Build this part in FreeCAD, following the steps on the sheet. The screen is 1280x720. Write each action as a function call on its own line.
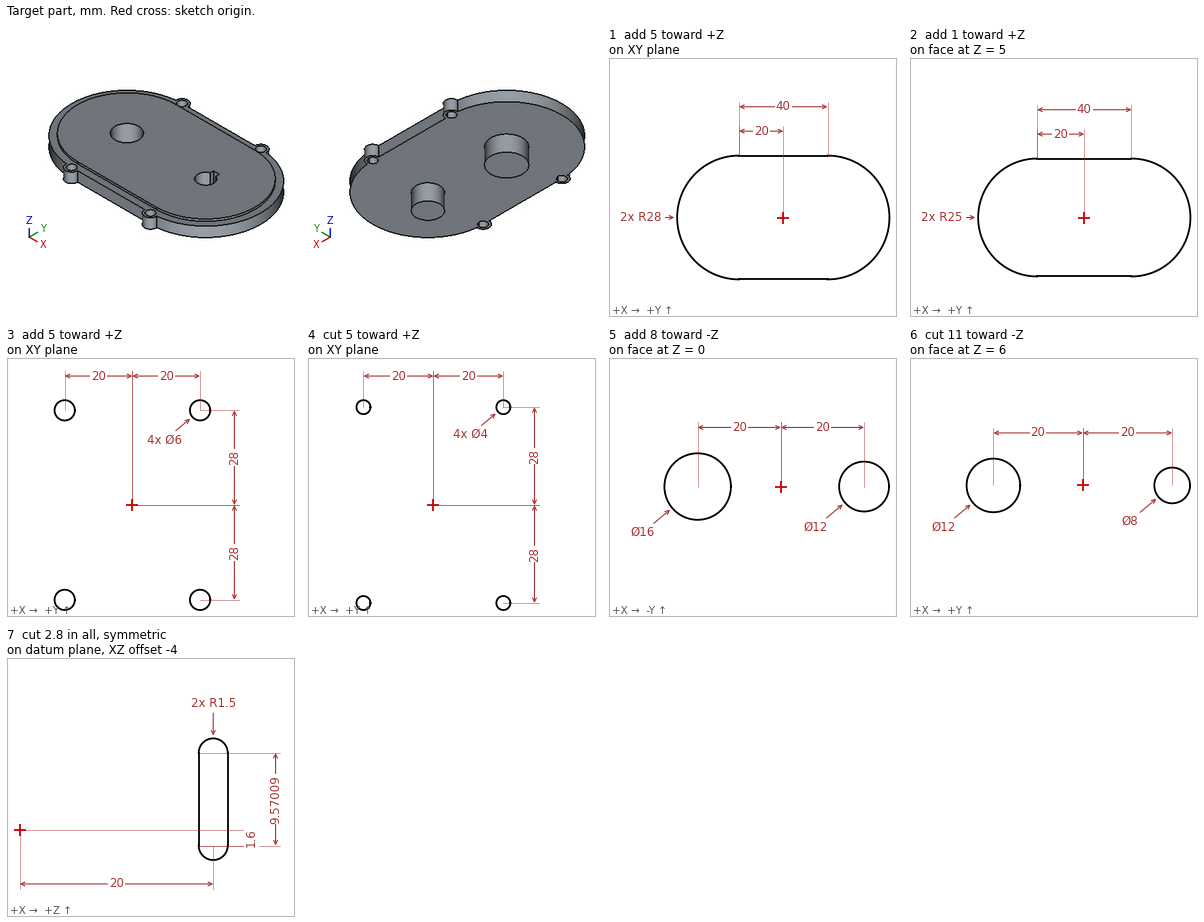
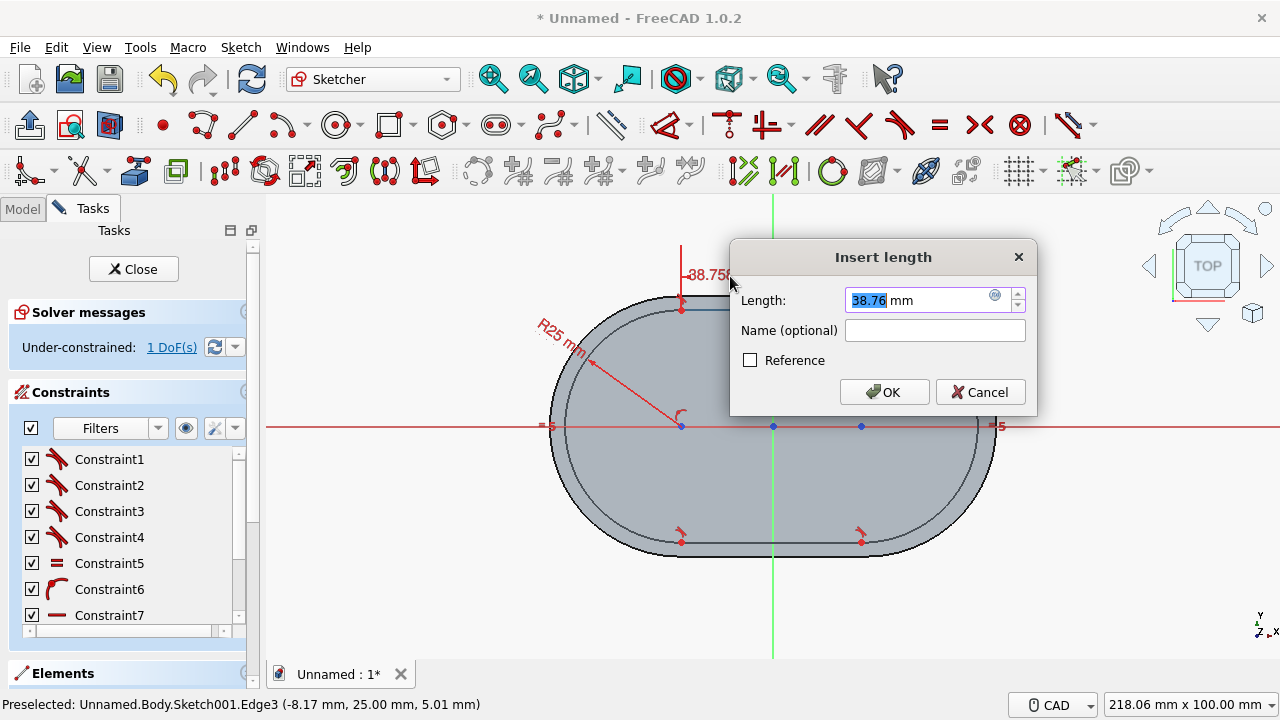
text(40)
key(Return)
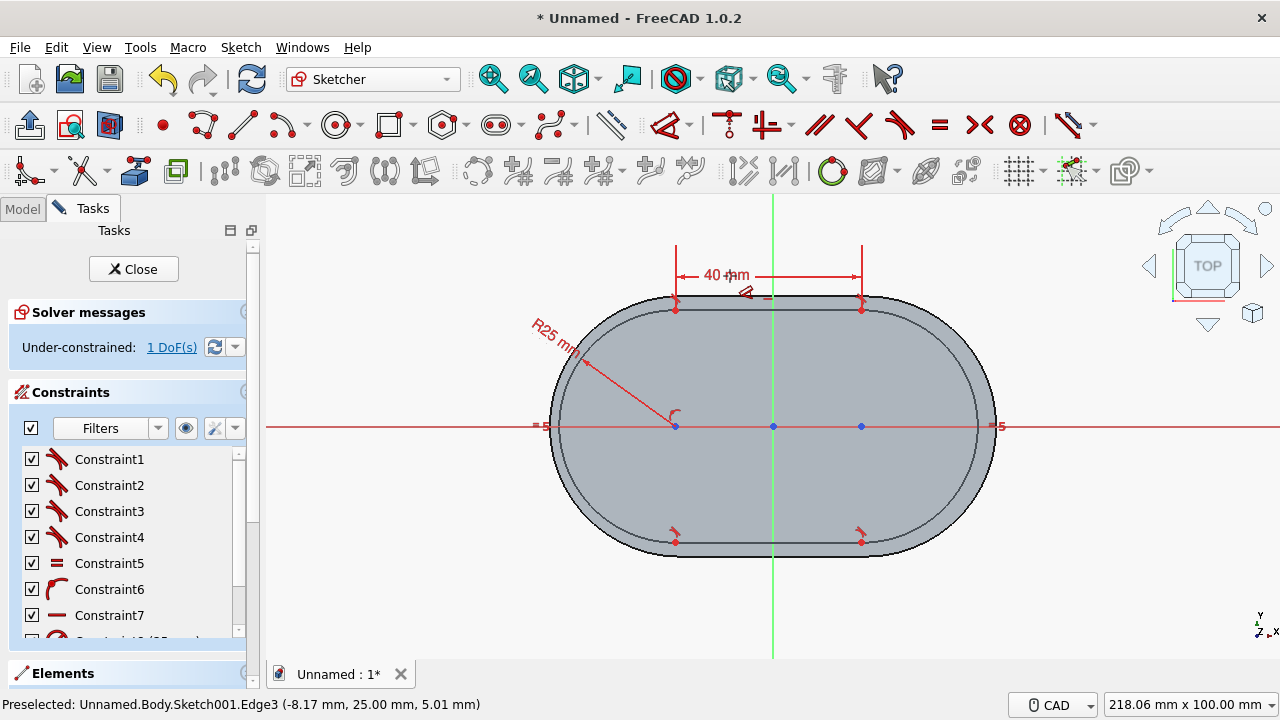
click(676, 310)
click(724, 460)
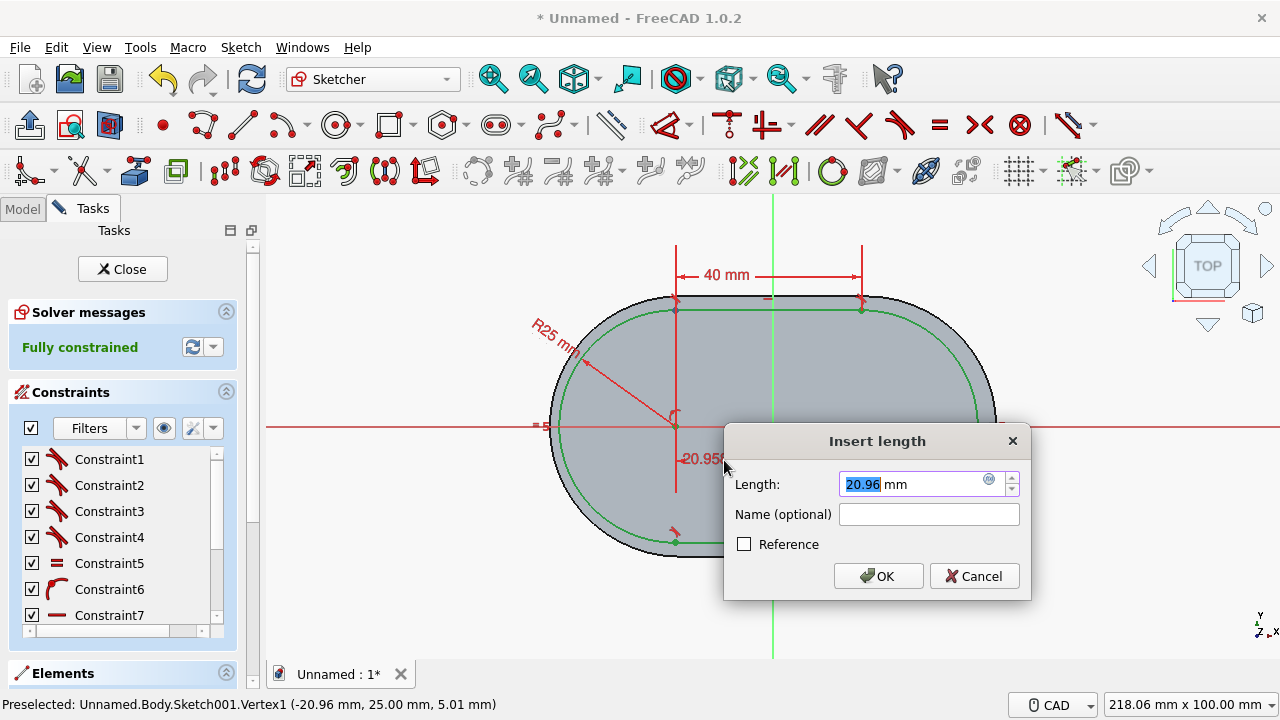
text(20)
key(Return)
key(Escape)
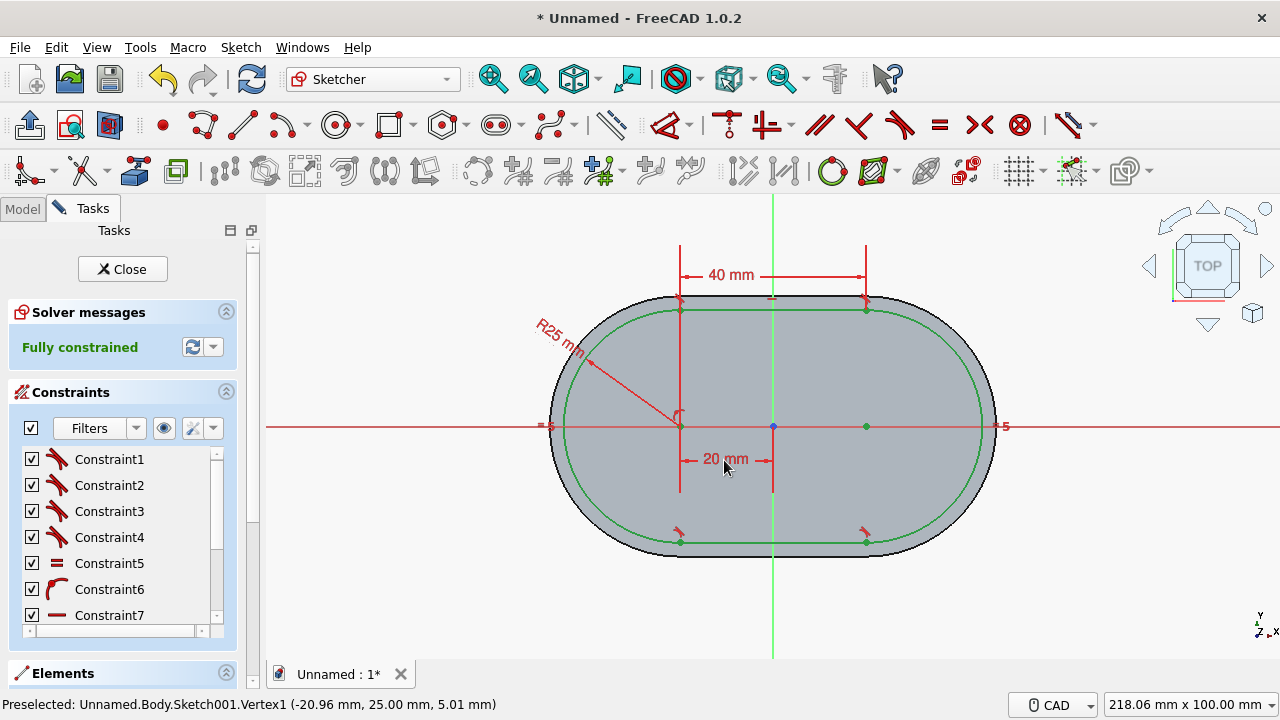
click(123, 269)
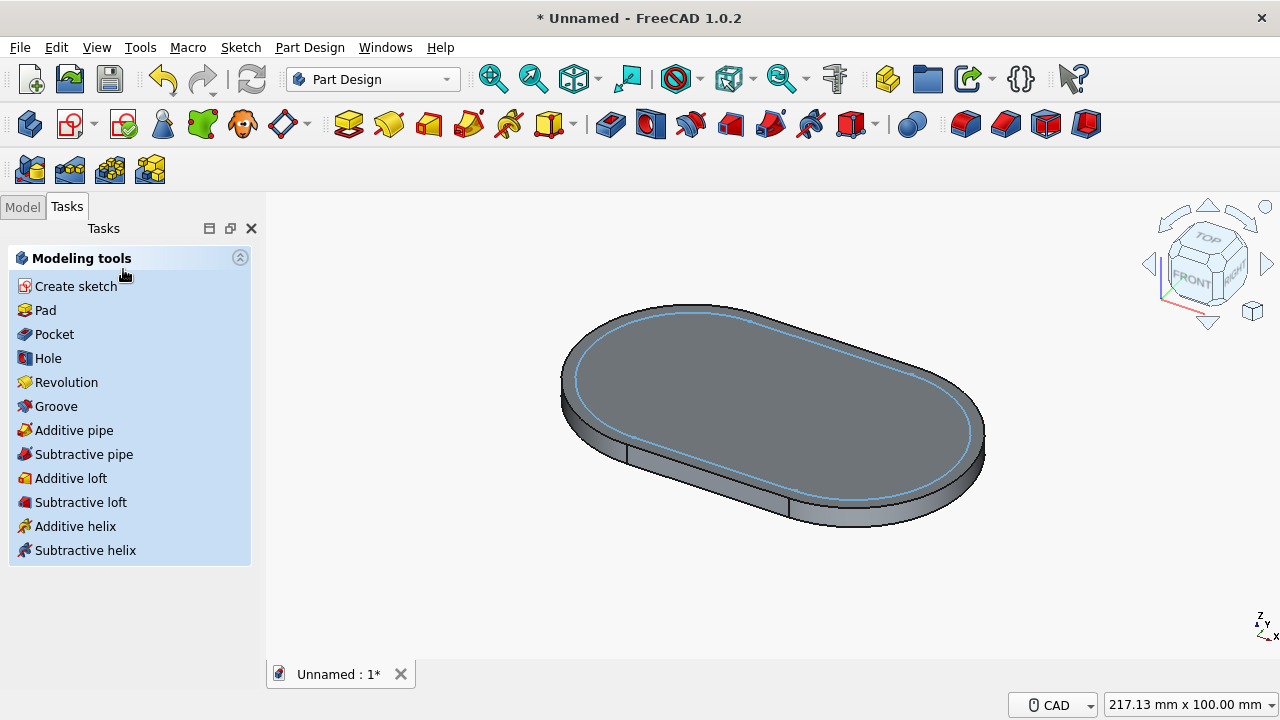
click(350, 124)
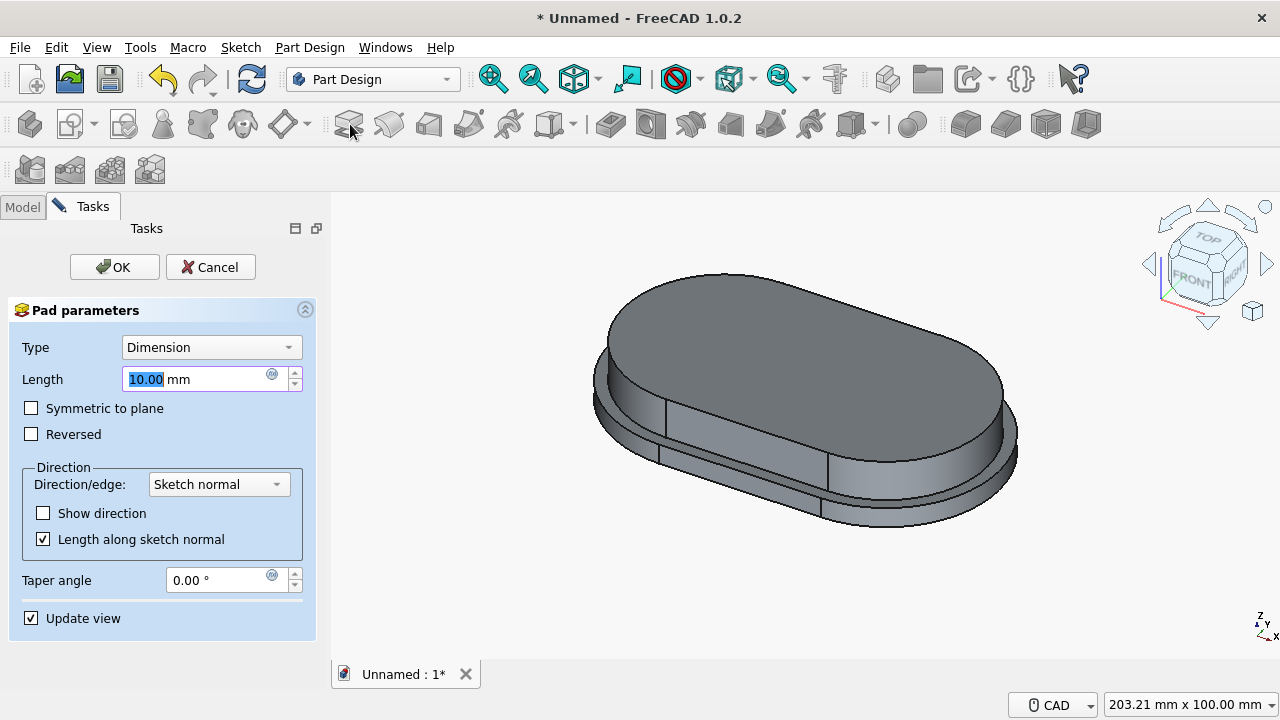
text(1)
key(Tab)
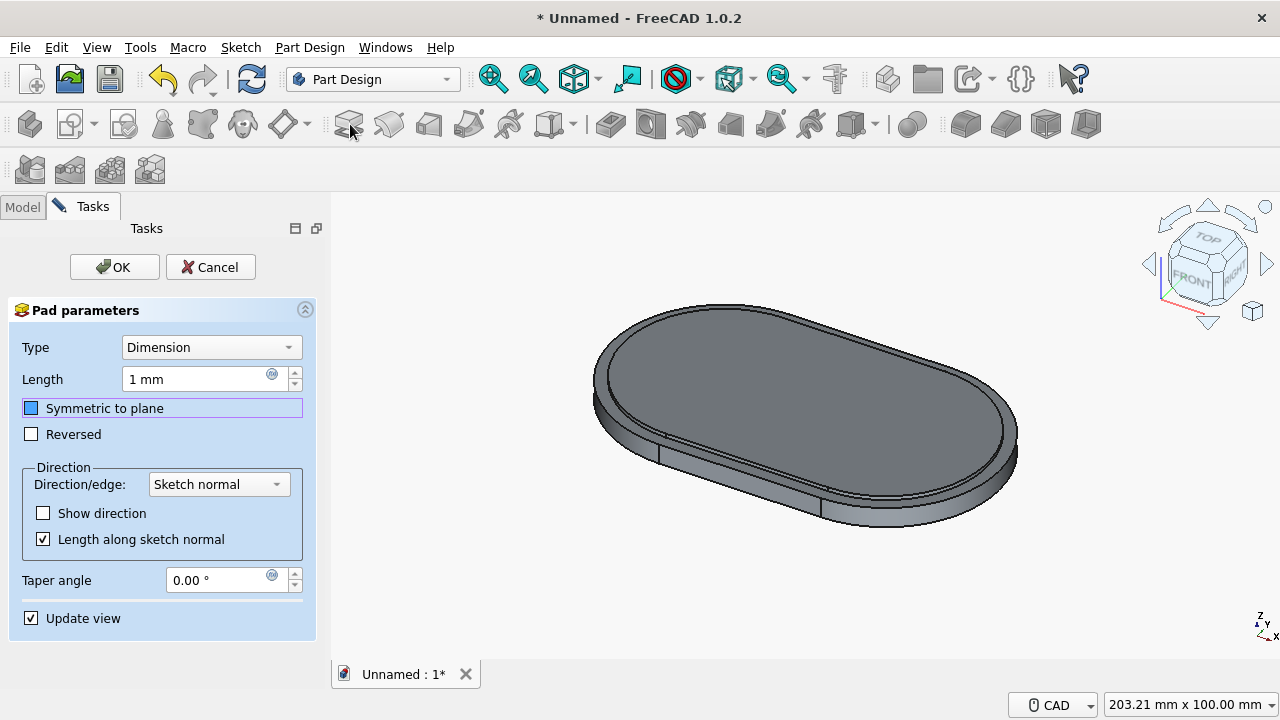
click(115, 267)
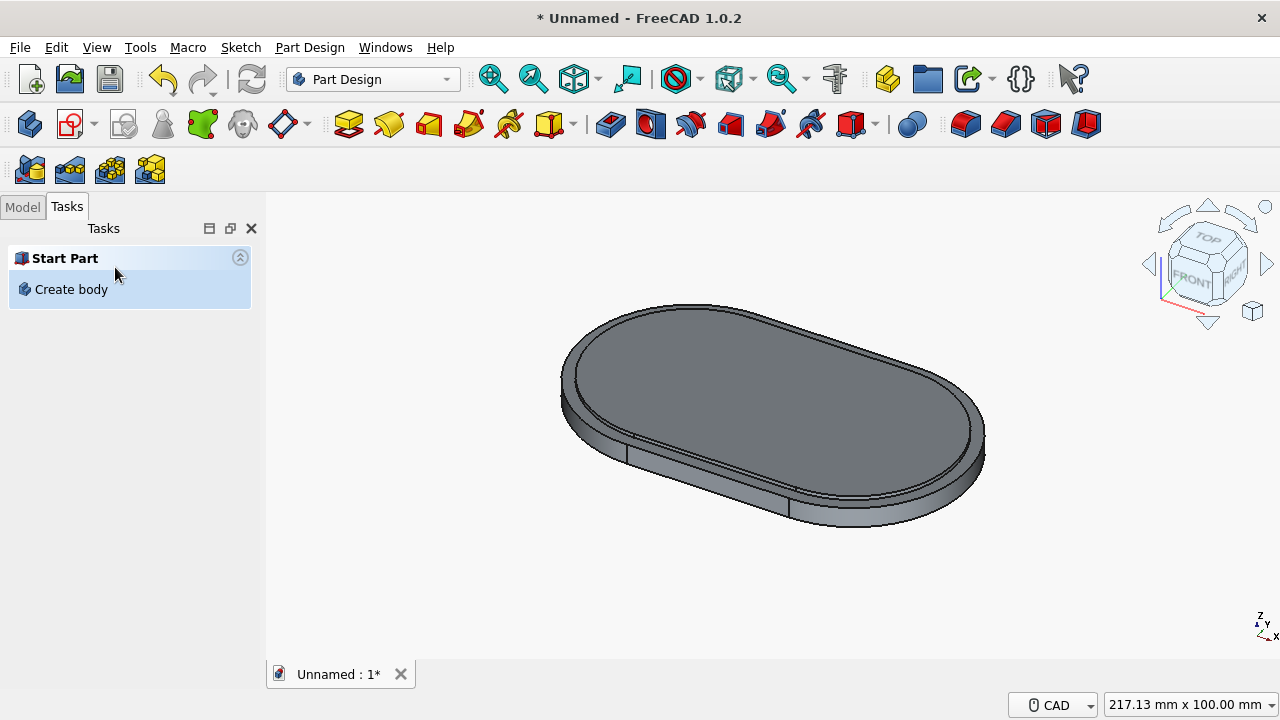
click(70, 124)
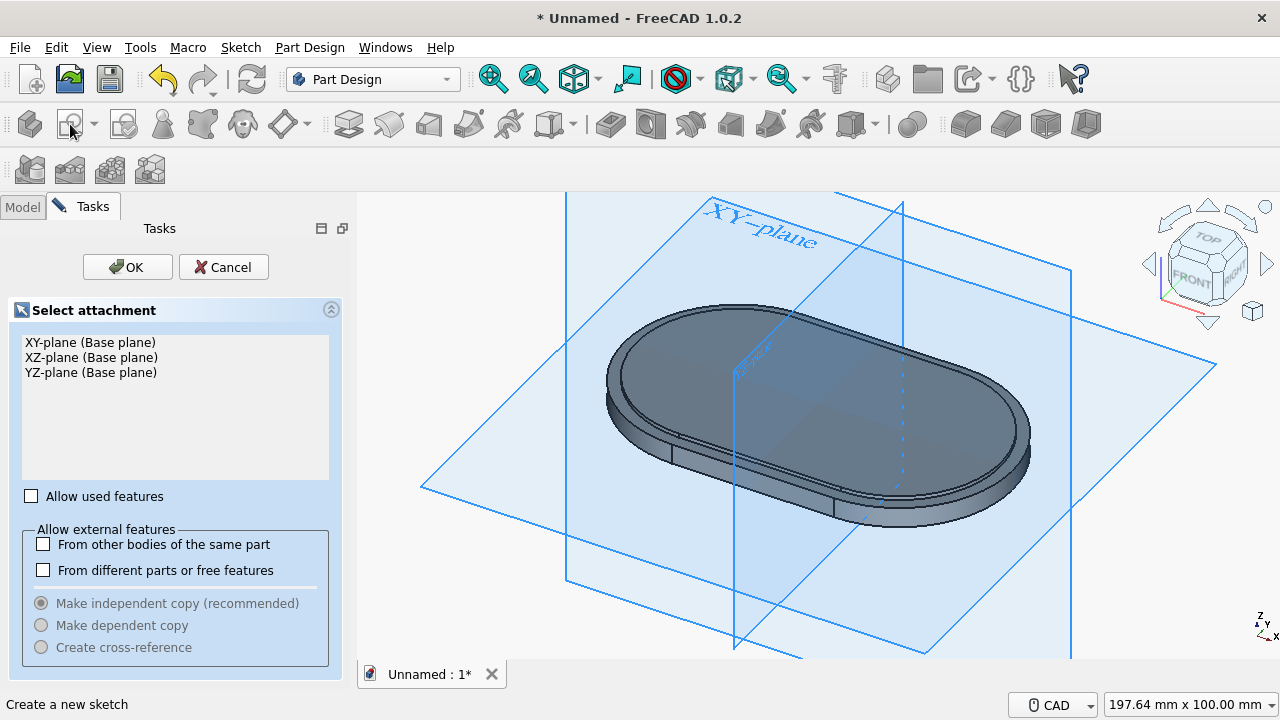
click(82, 342)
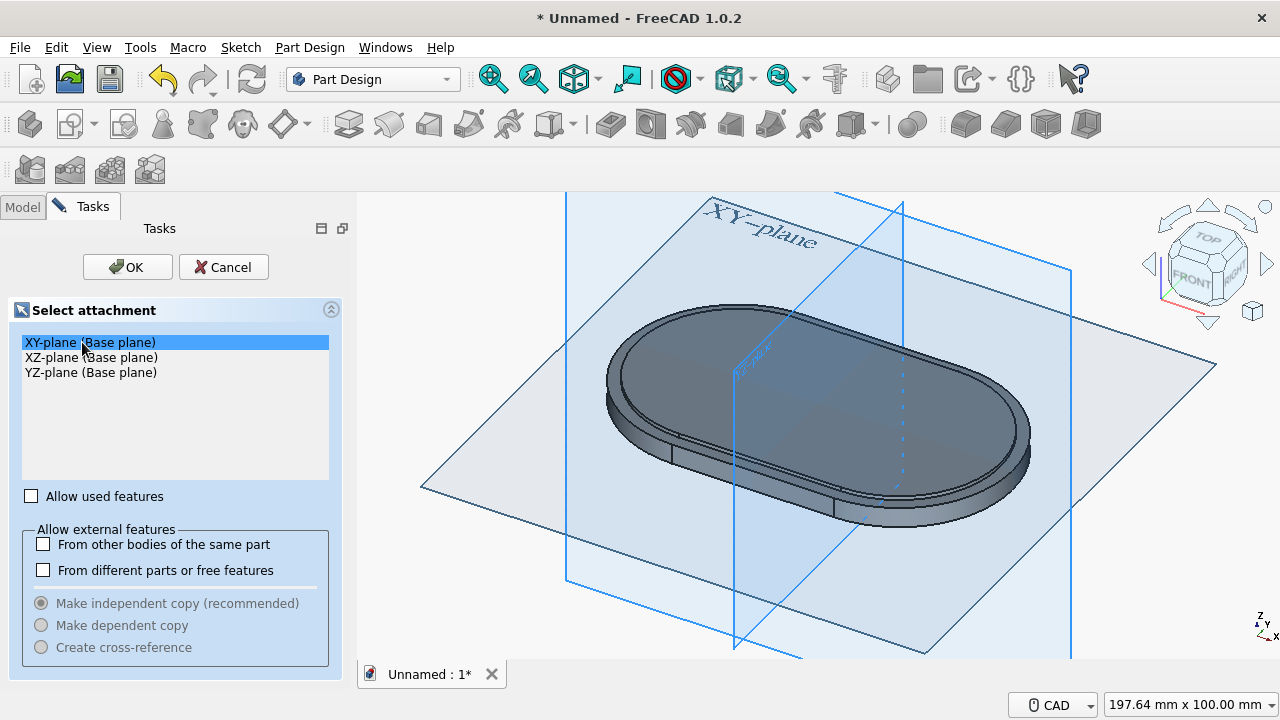
click(128, 267)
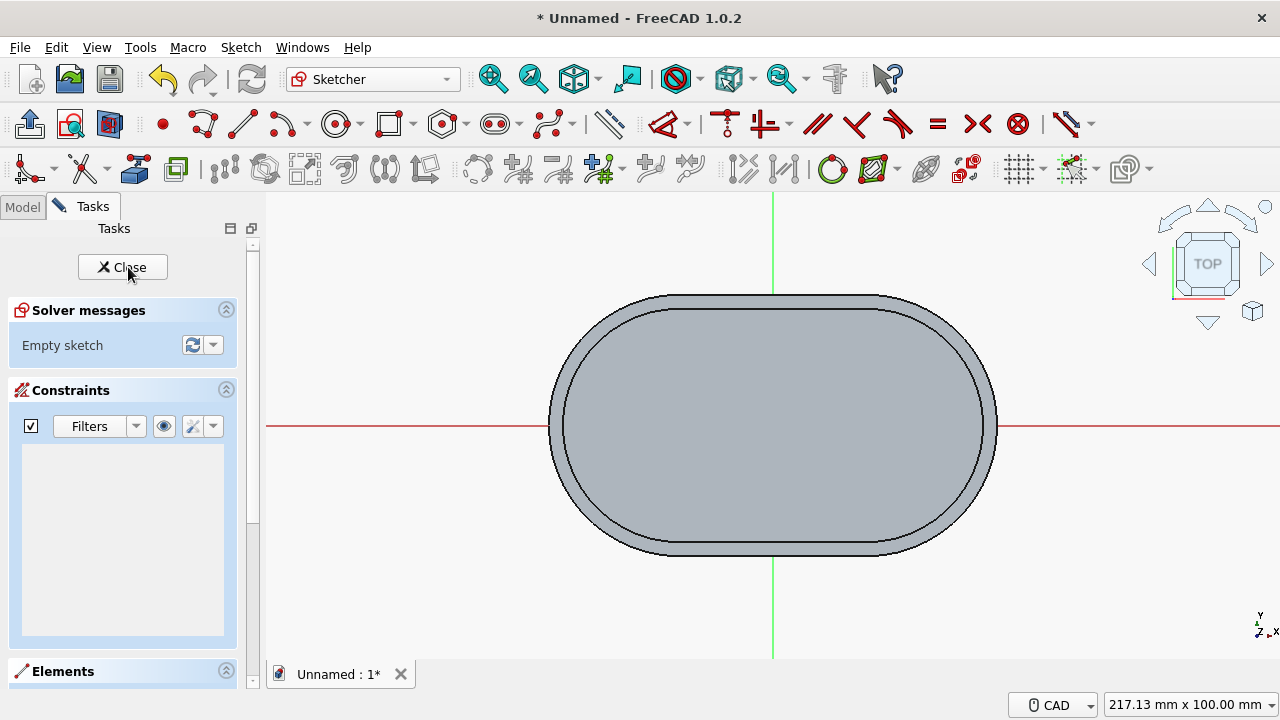
key(q)
key(s)